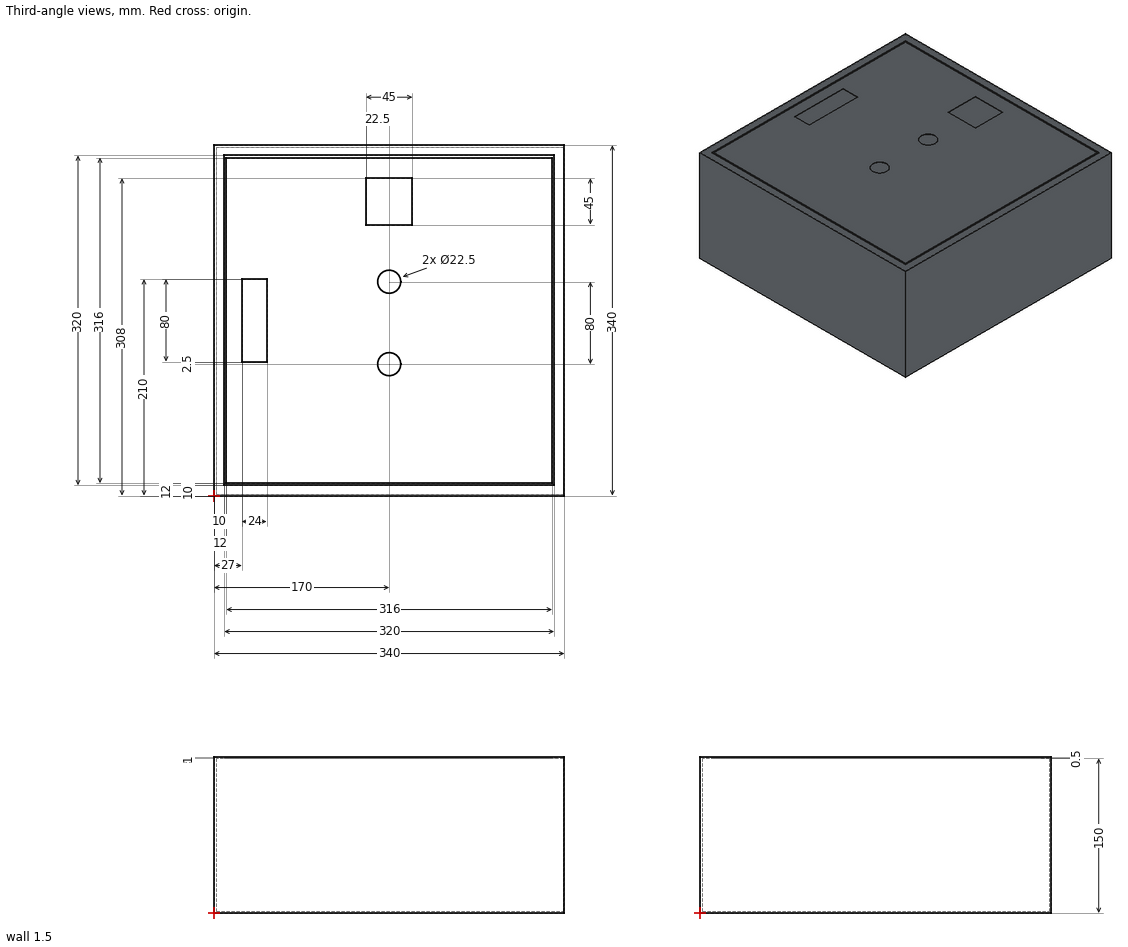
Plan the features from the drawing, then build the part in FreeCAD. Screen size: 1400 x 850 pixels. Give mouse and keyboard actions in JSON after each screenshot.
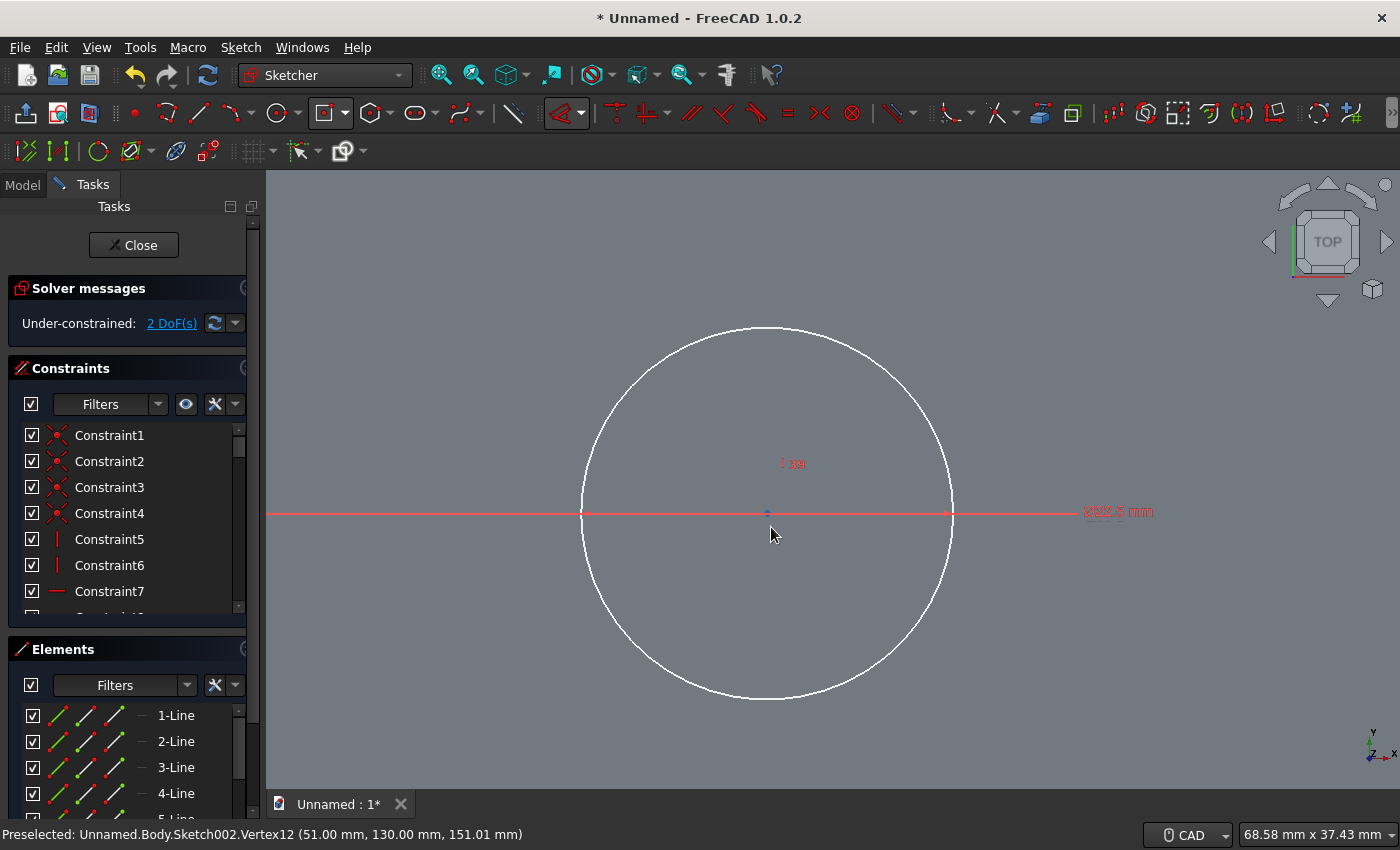
{"action": "left_click", "coordinate": [767, 514]}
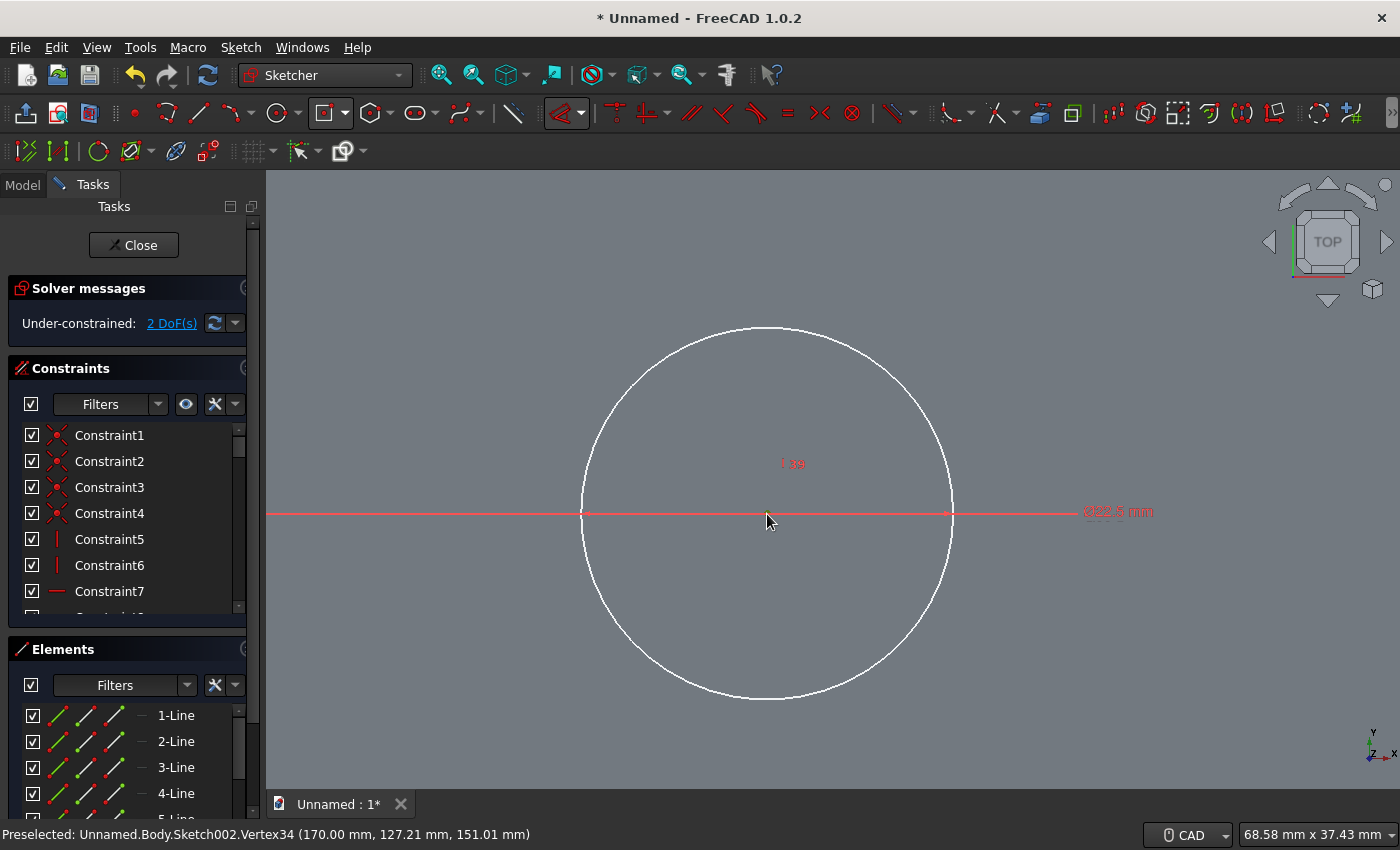
{"action": "key", "text": "i"}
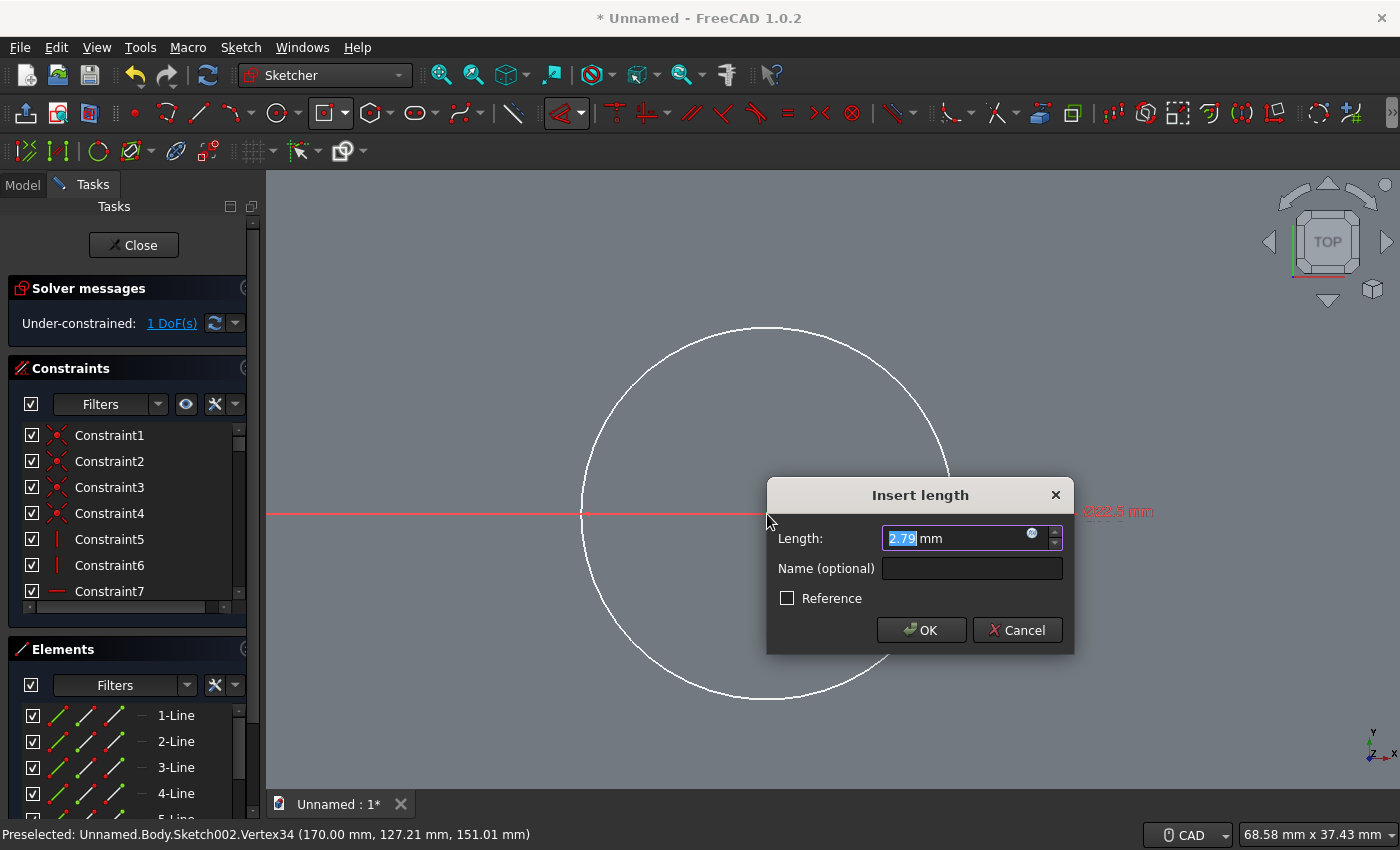
{"action": "type", "text": "2.5"}
{"action": "key", "text": "Return"}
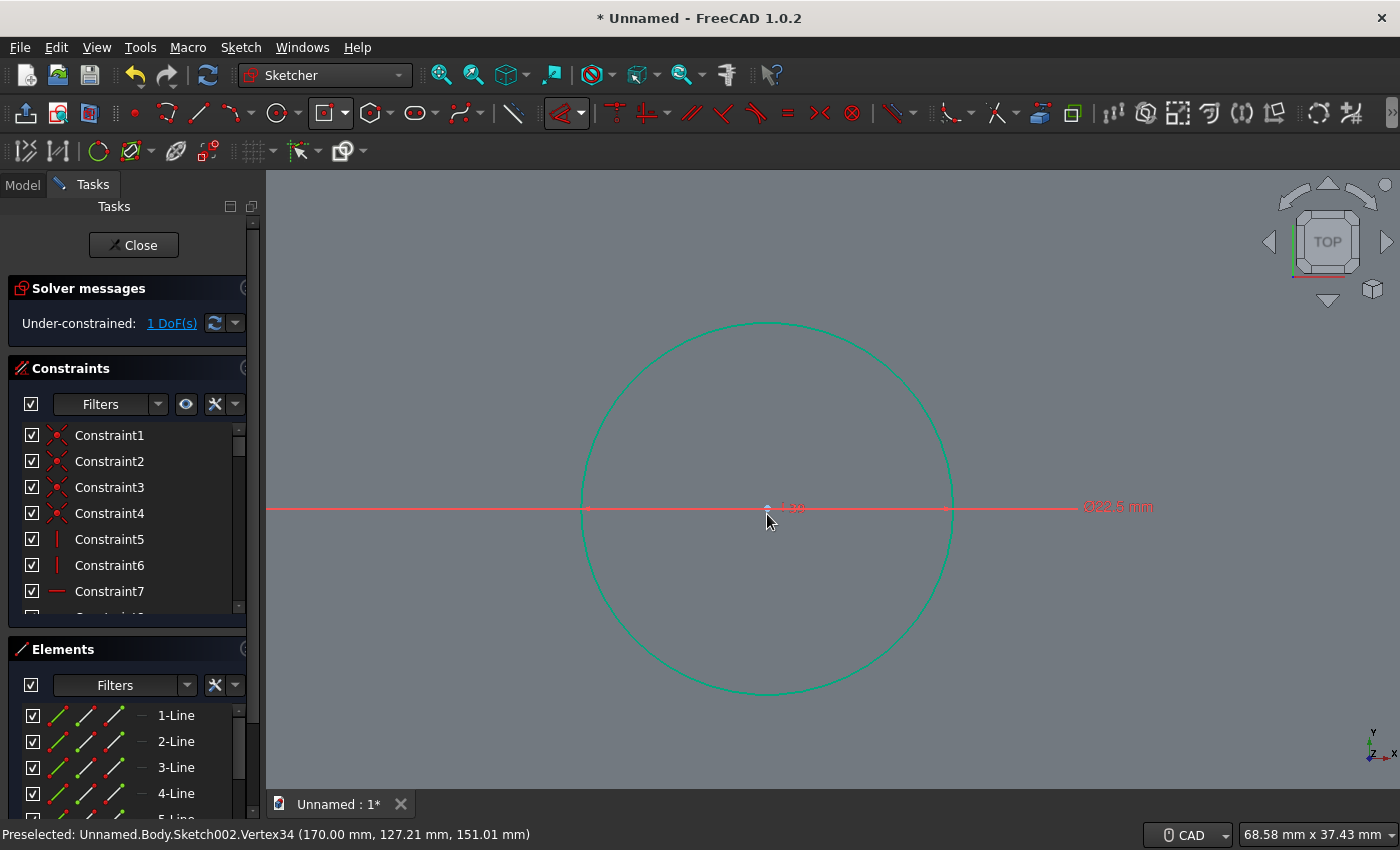
{"action": "scroll", "coordinate": [771, 527], "scroll_direction": "down", "scroll_amount": 13}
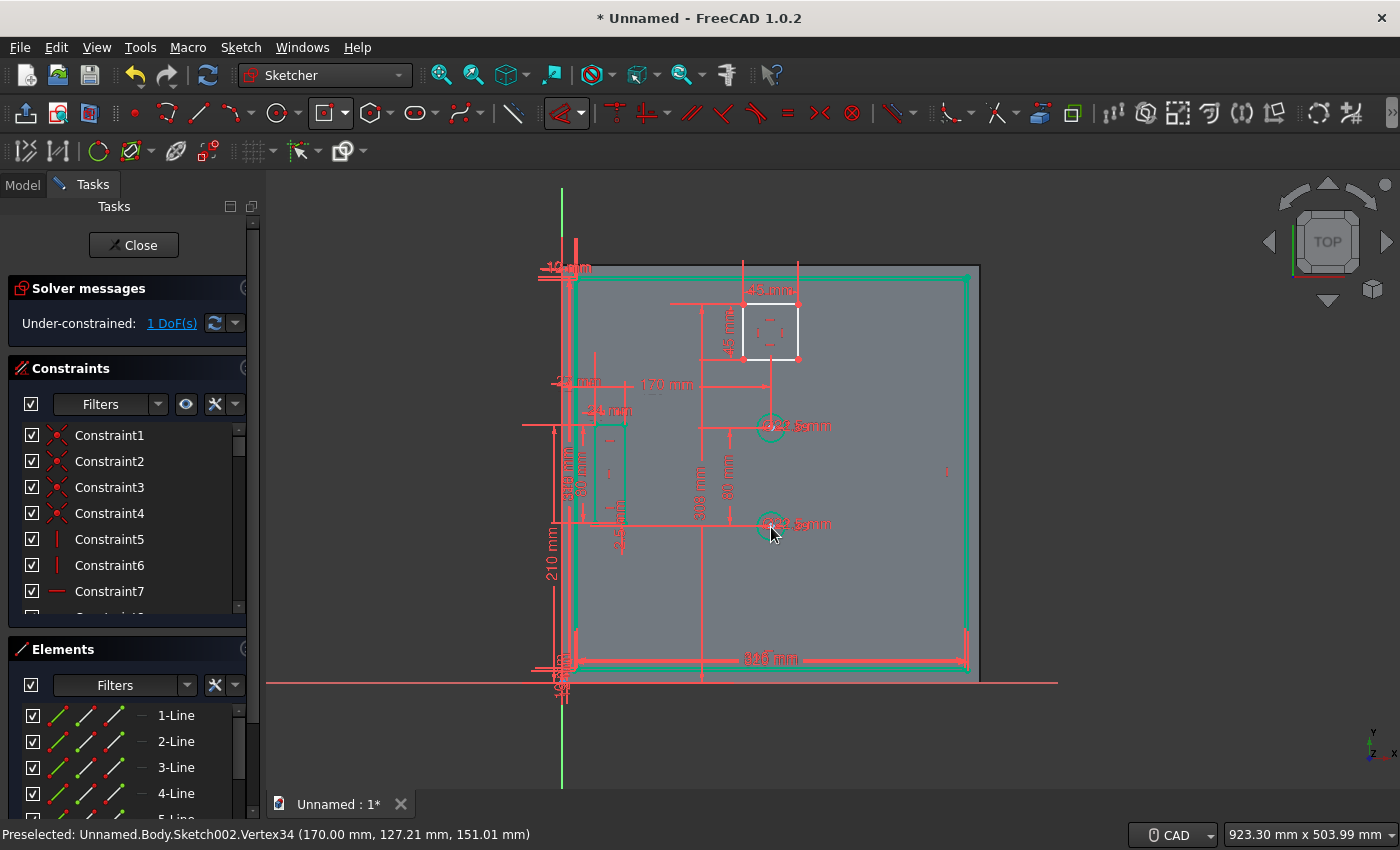
{"action": "scroll", "coordinate": [743, 360], "scroll_direction": "up", "scroll_amount": 2}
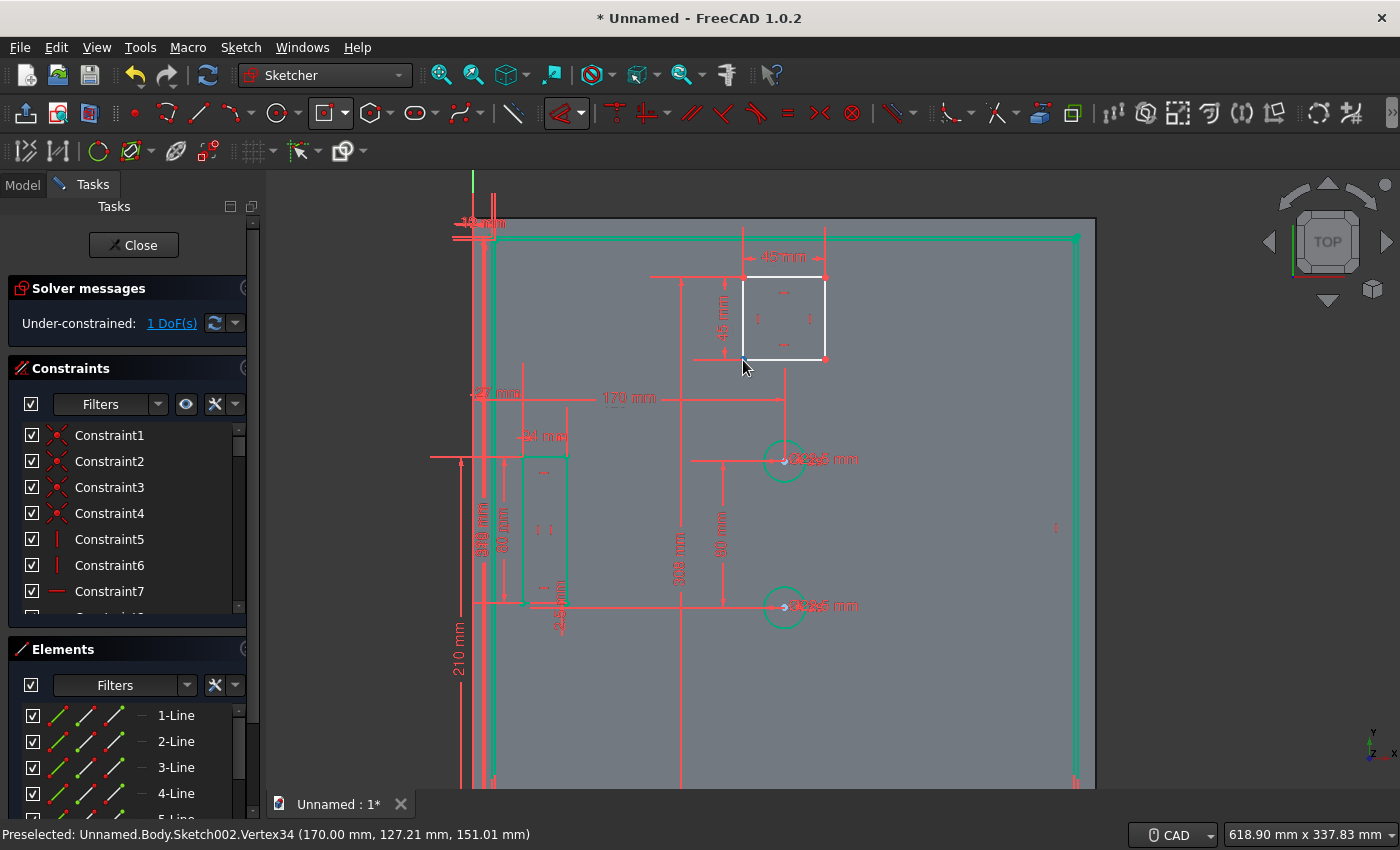
{"action": "left_click", "coordinate": [743, 360]}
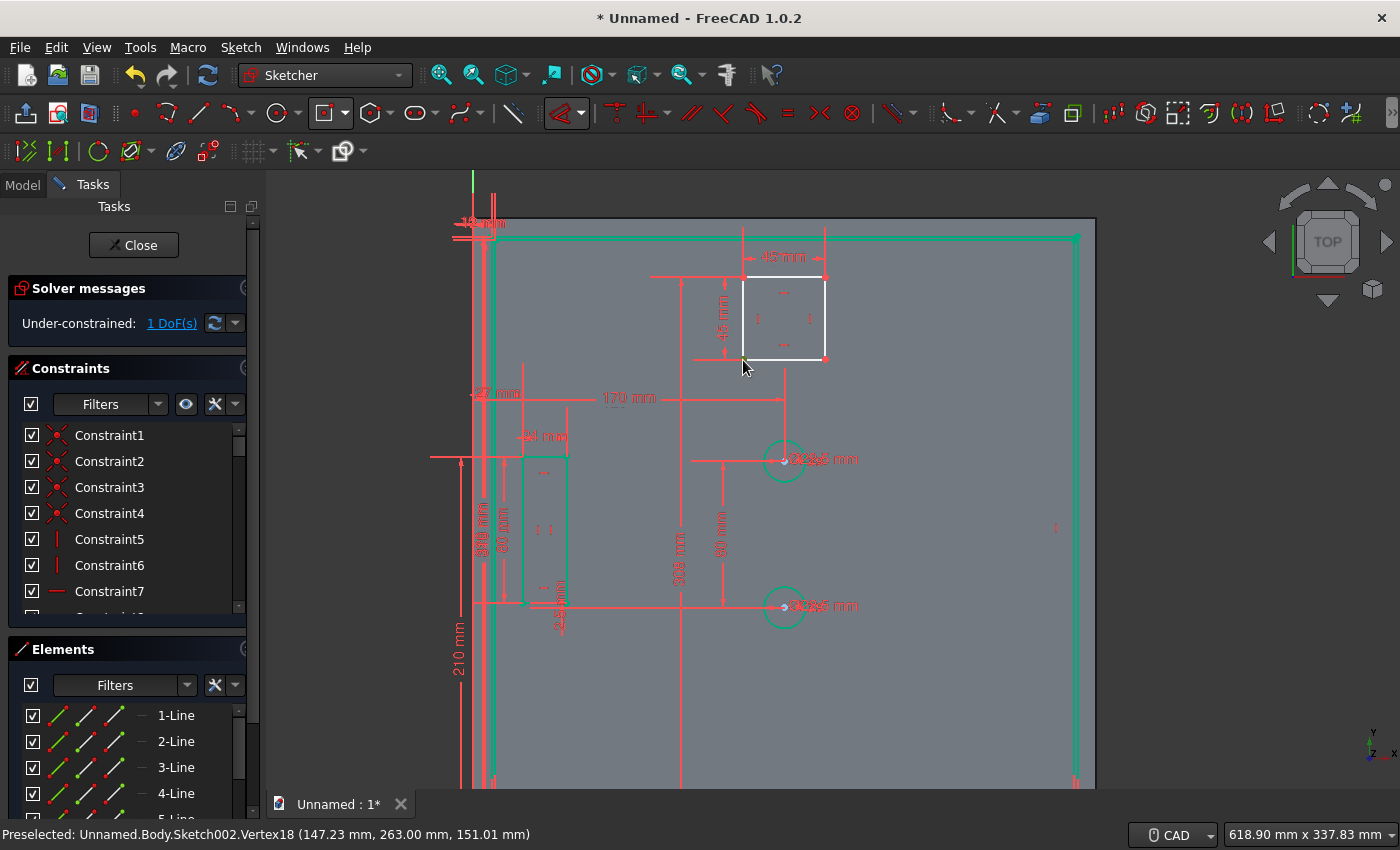
{"action": "left_click", "coordinate": [785, 461]}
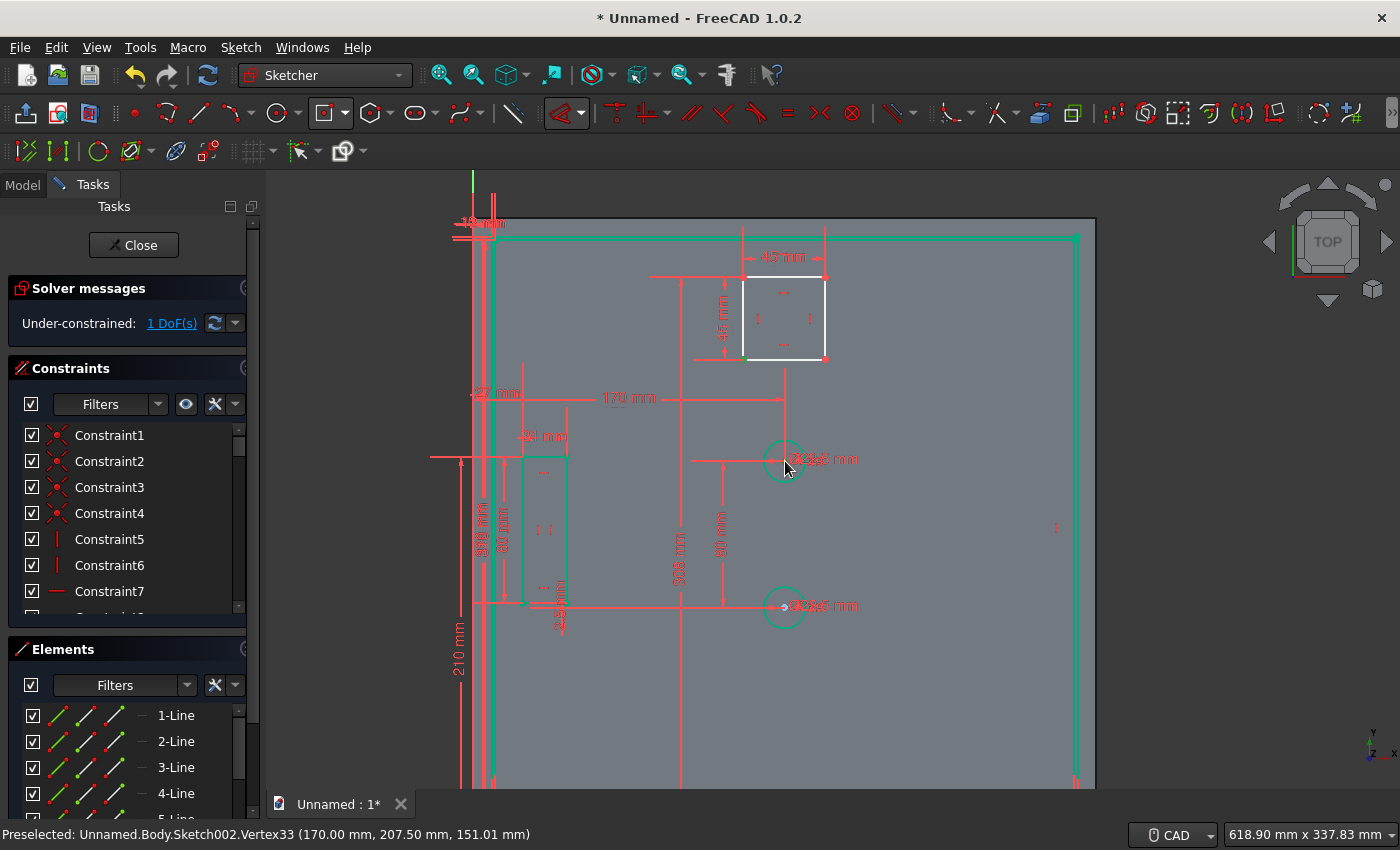
{"action": "key", "text": "l"}